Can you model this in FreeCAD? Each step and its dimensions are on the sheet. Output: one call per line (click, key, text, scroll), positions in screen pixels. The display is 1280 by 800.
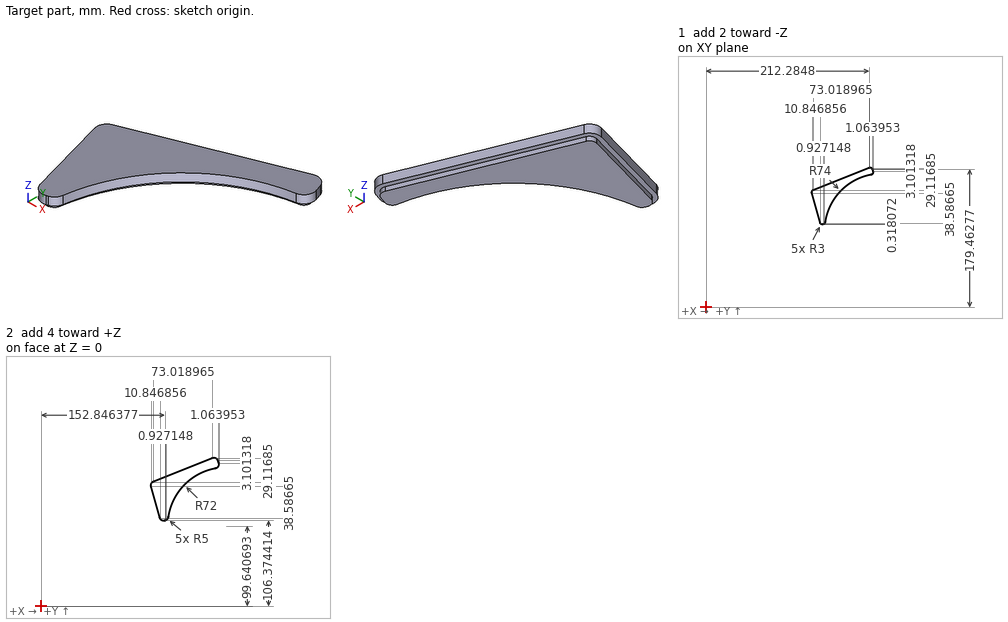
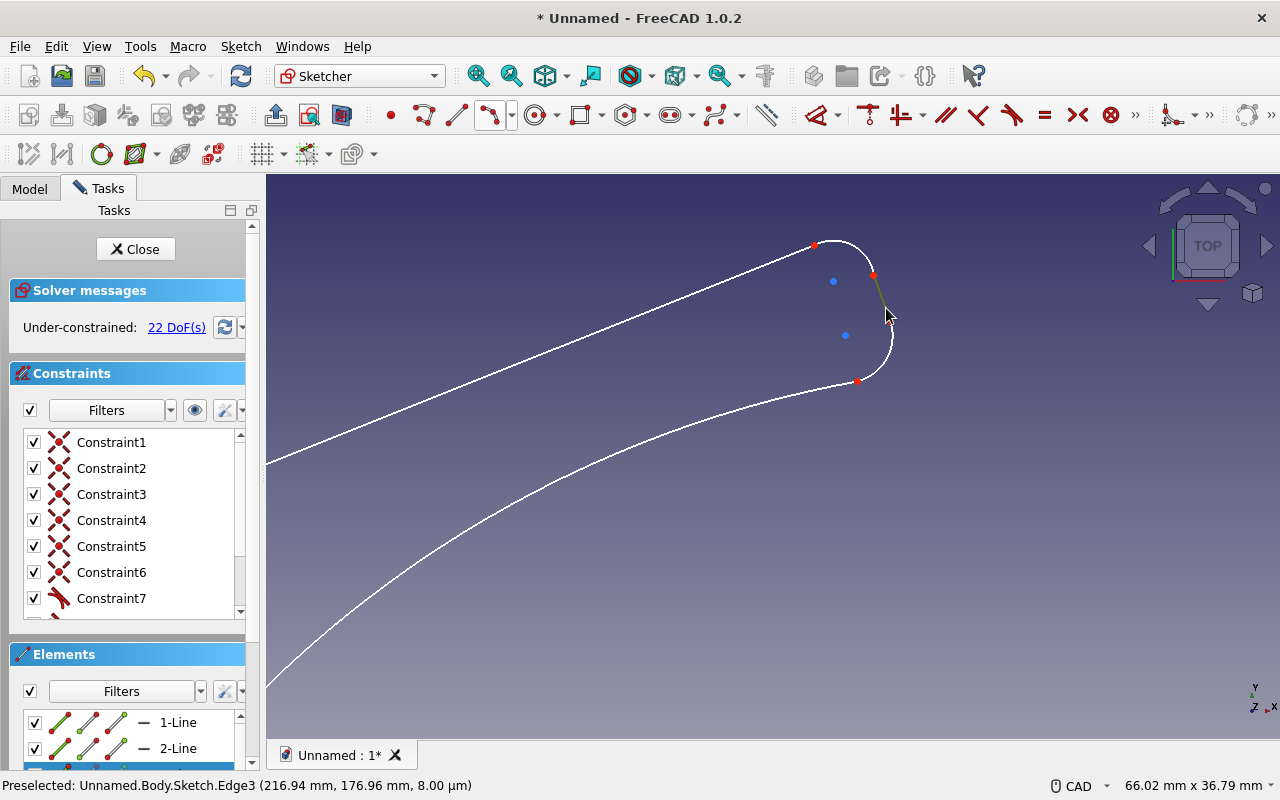
click(877, 371)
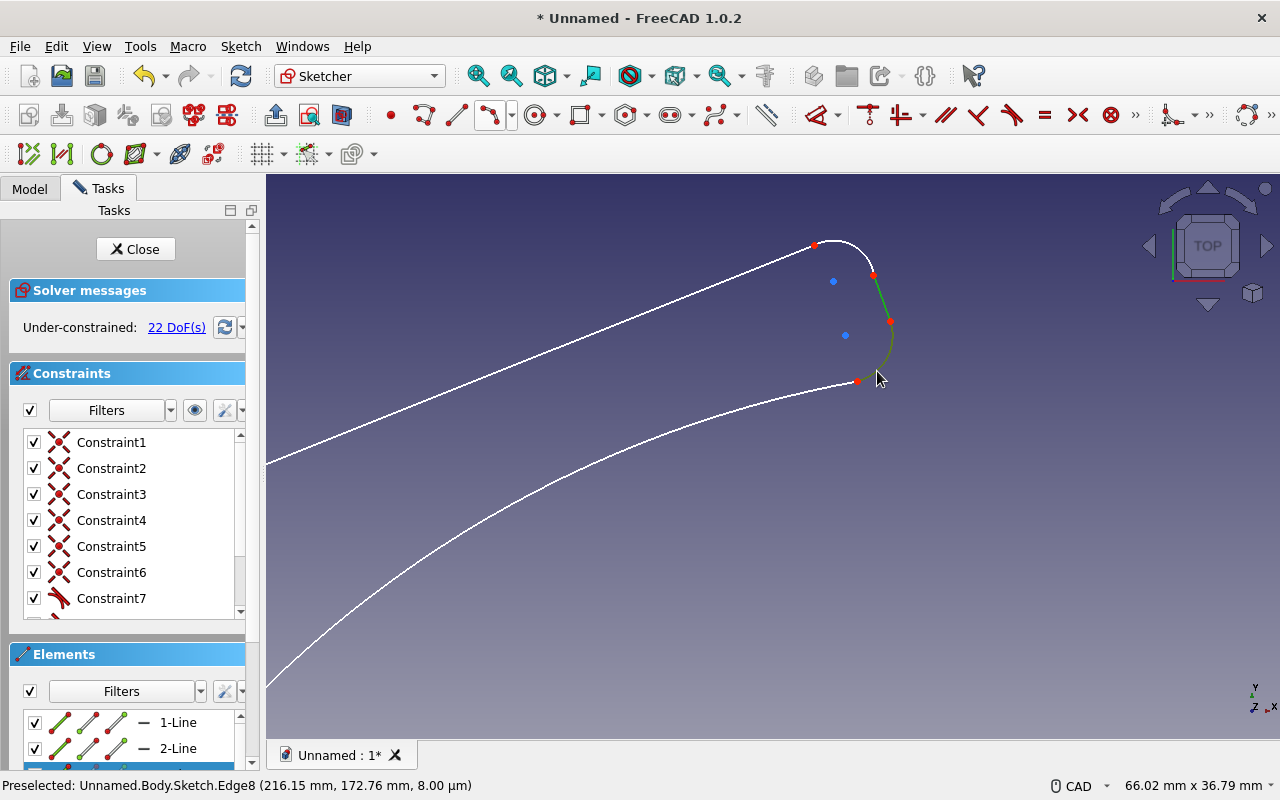
click(1012, 116)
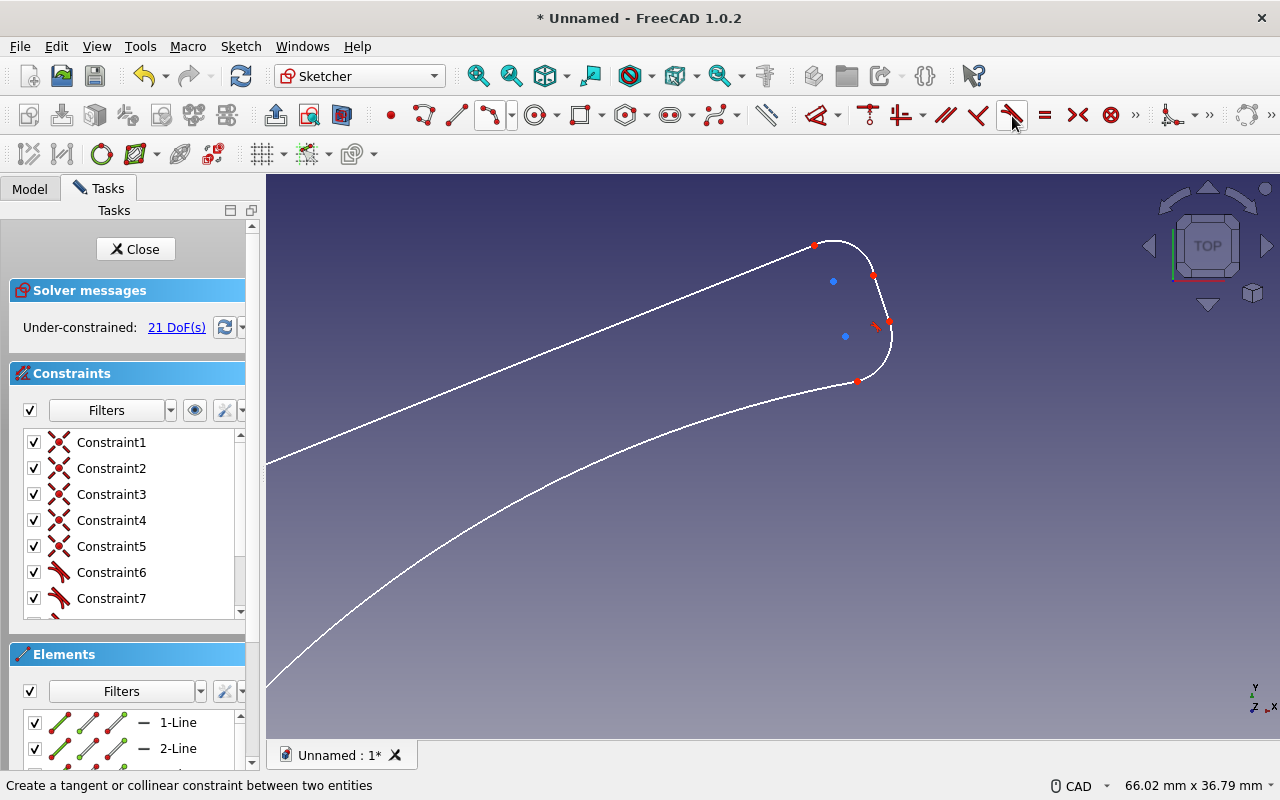
click(885, 308)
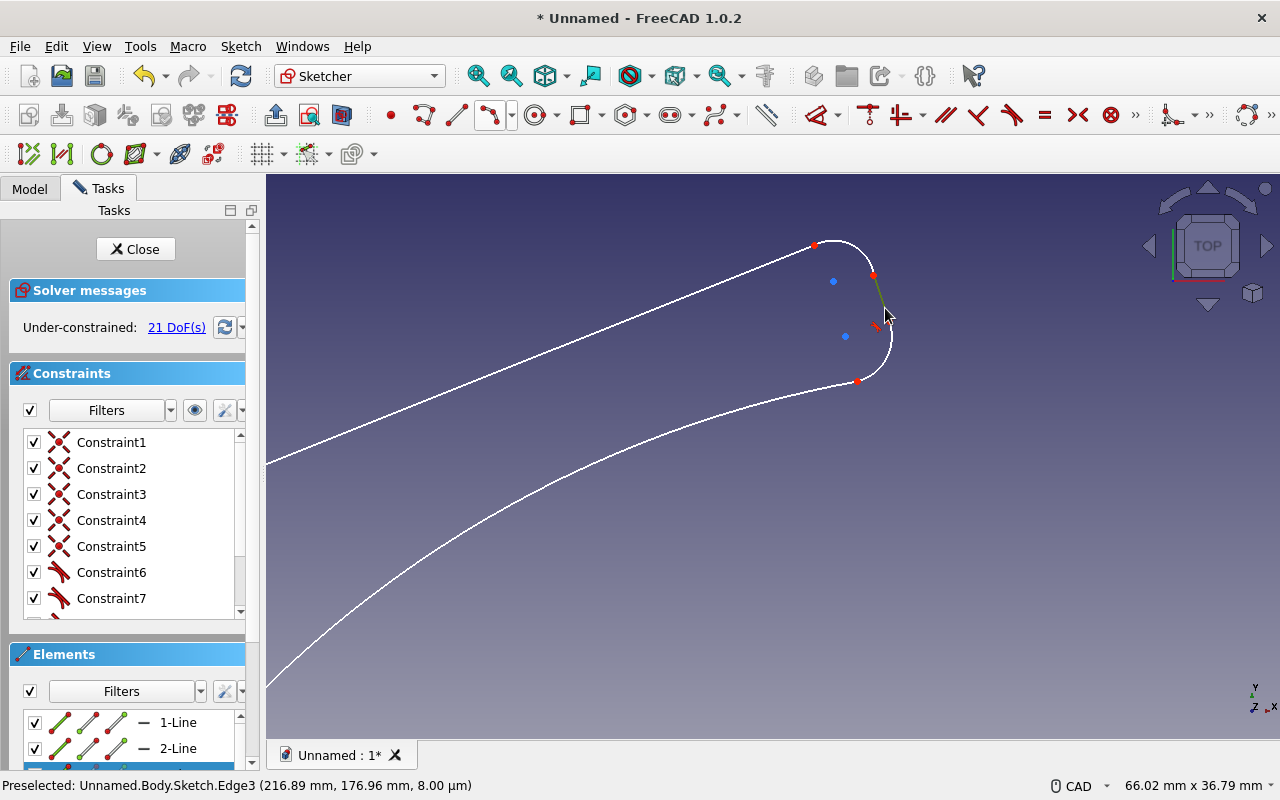
click(864, 254)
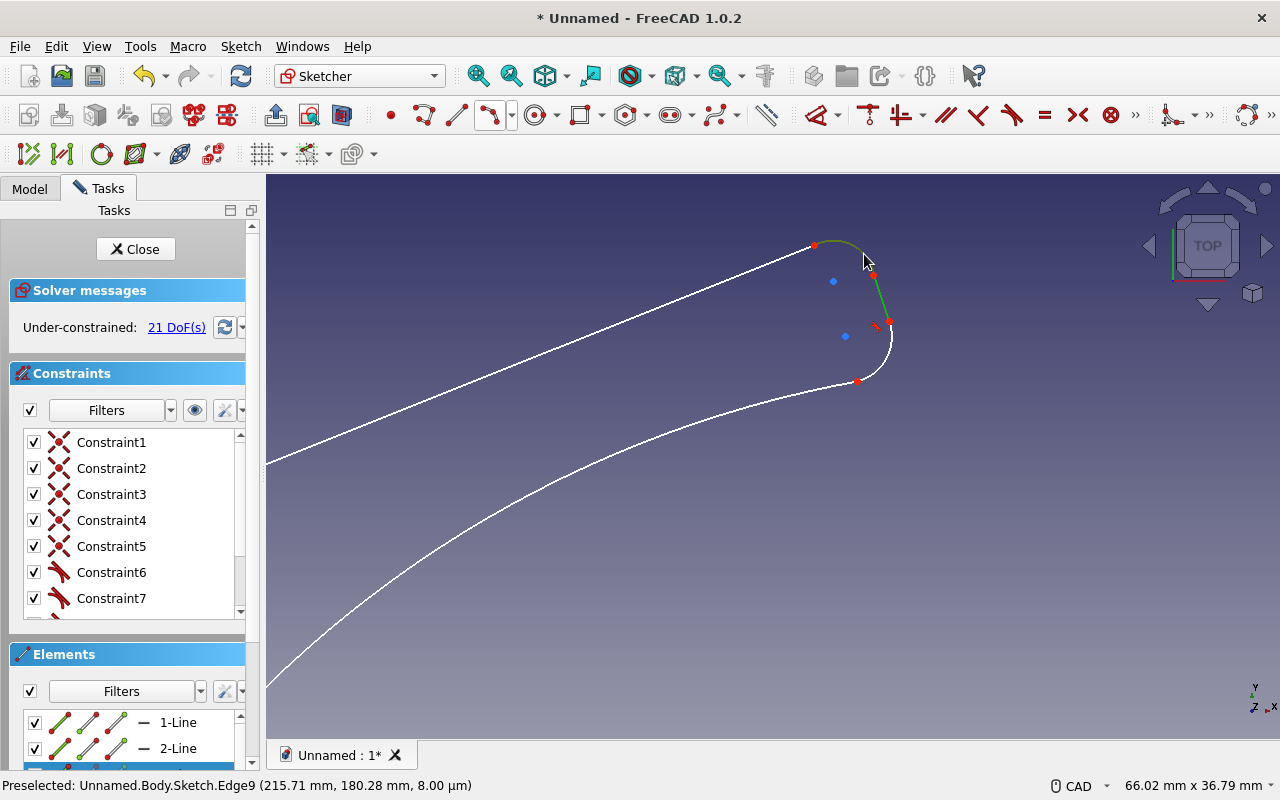
click(1012, 116)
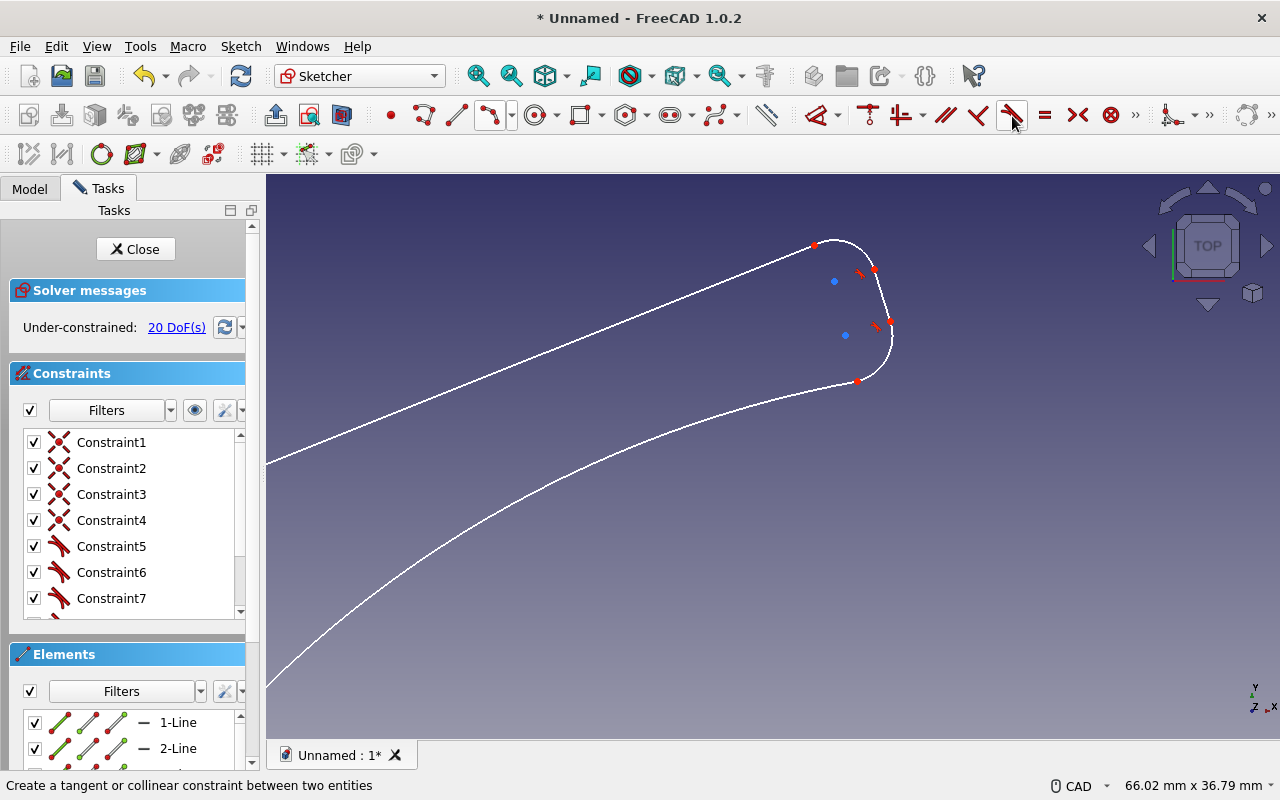
click(477, 380)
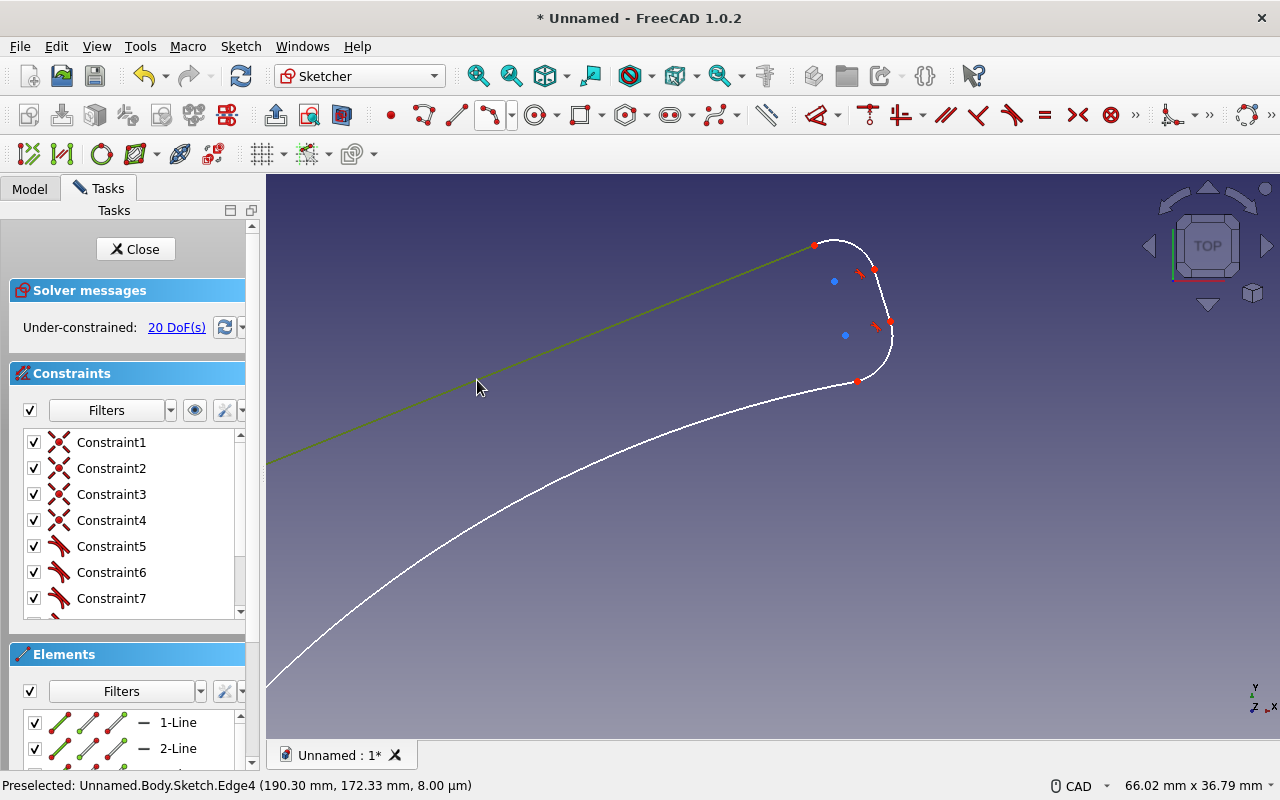
click(862, 251)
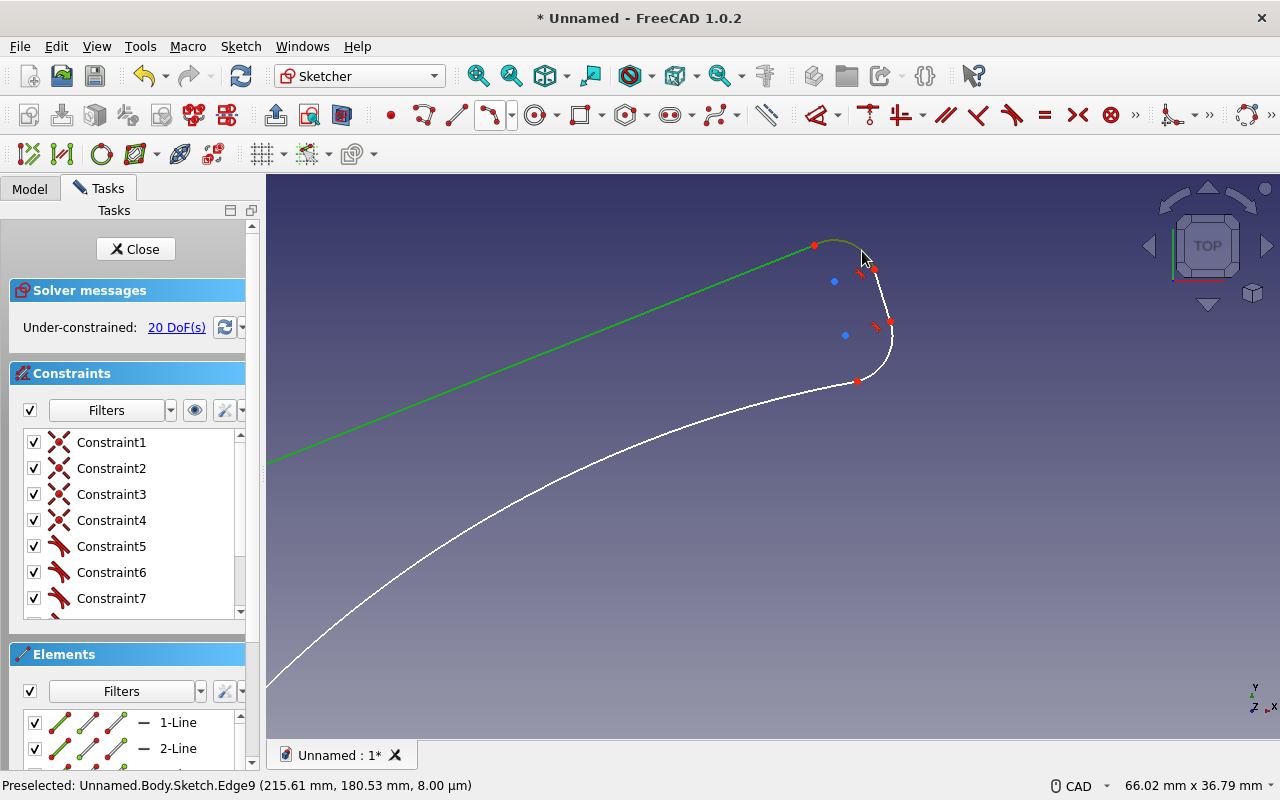
click(1012, 116)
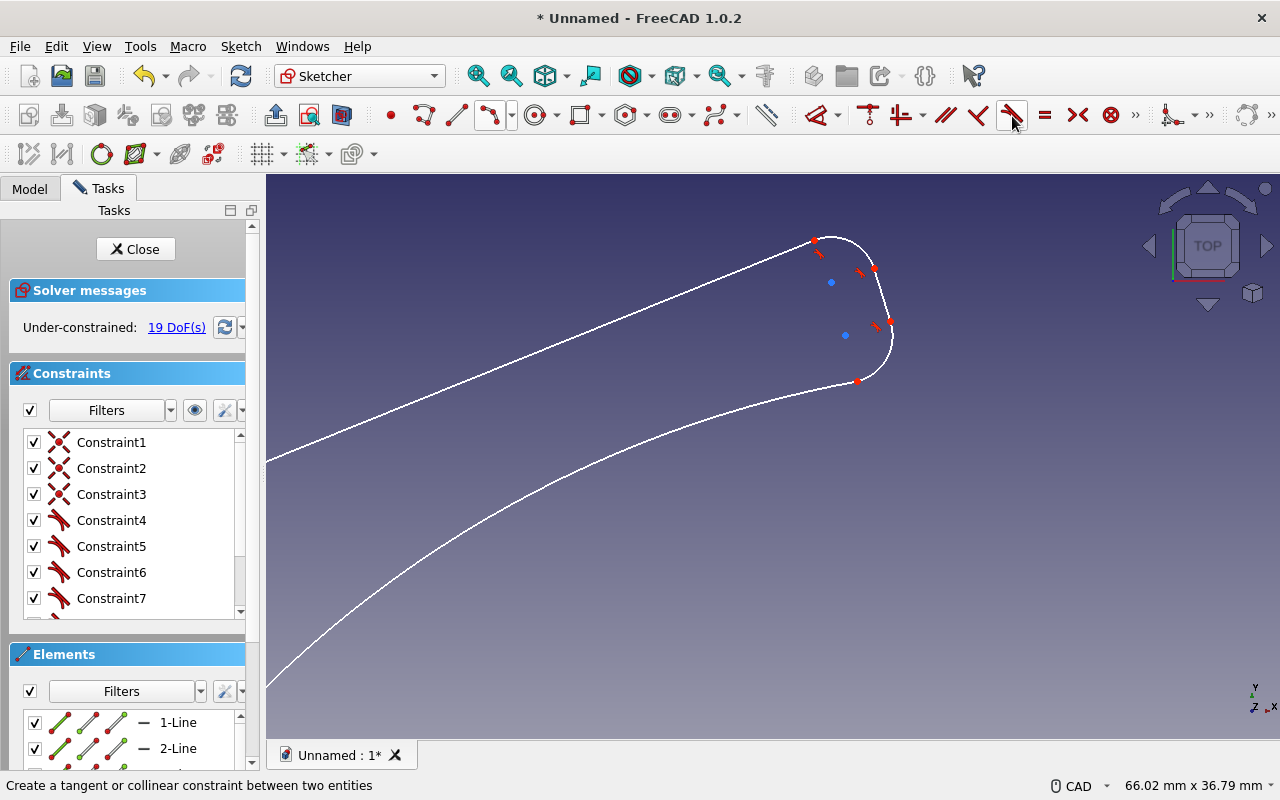
click(478, 376)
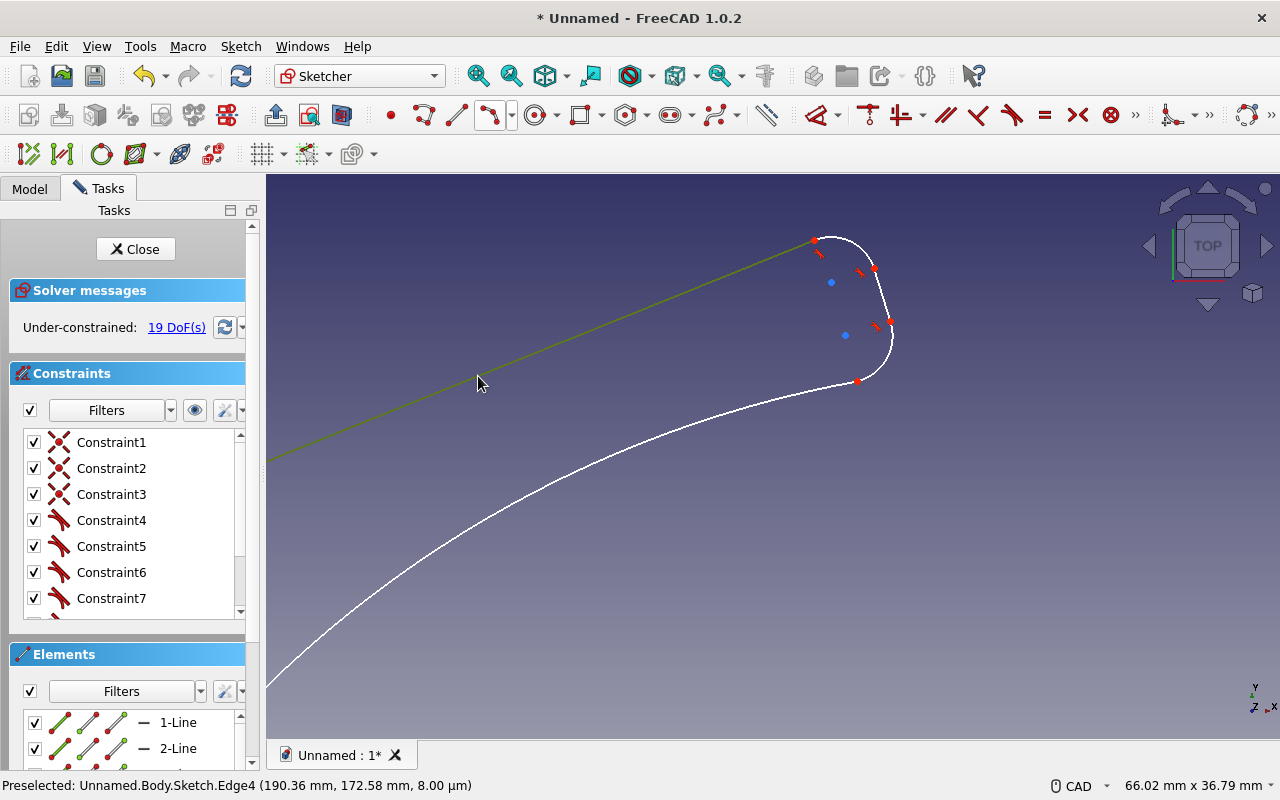
scroll(888, 306, down, 6)